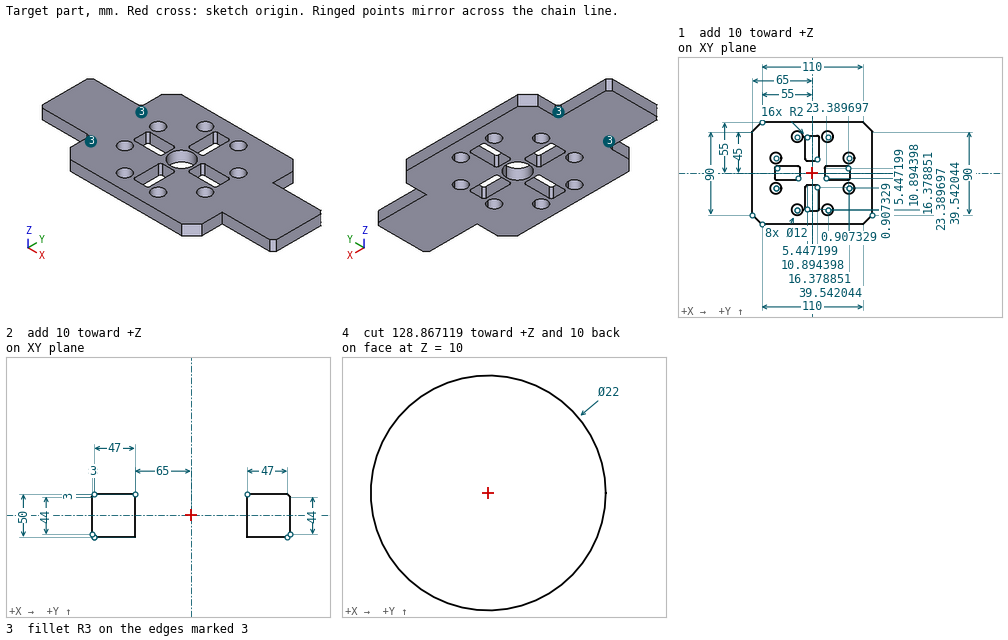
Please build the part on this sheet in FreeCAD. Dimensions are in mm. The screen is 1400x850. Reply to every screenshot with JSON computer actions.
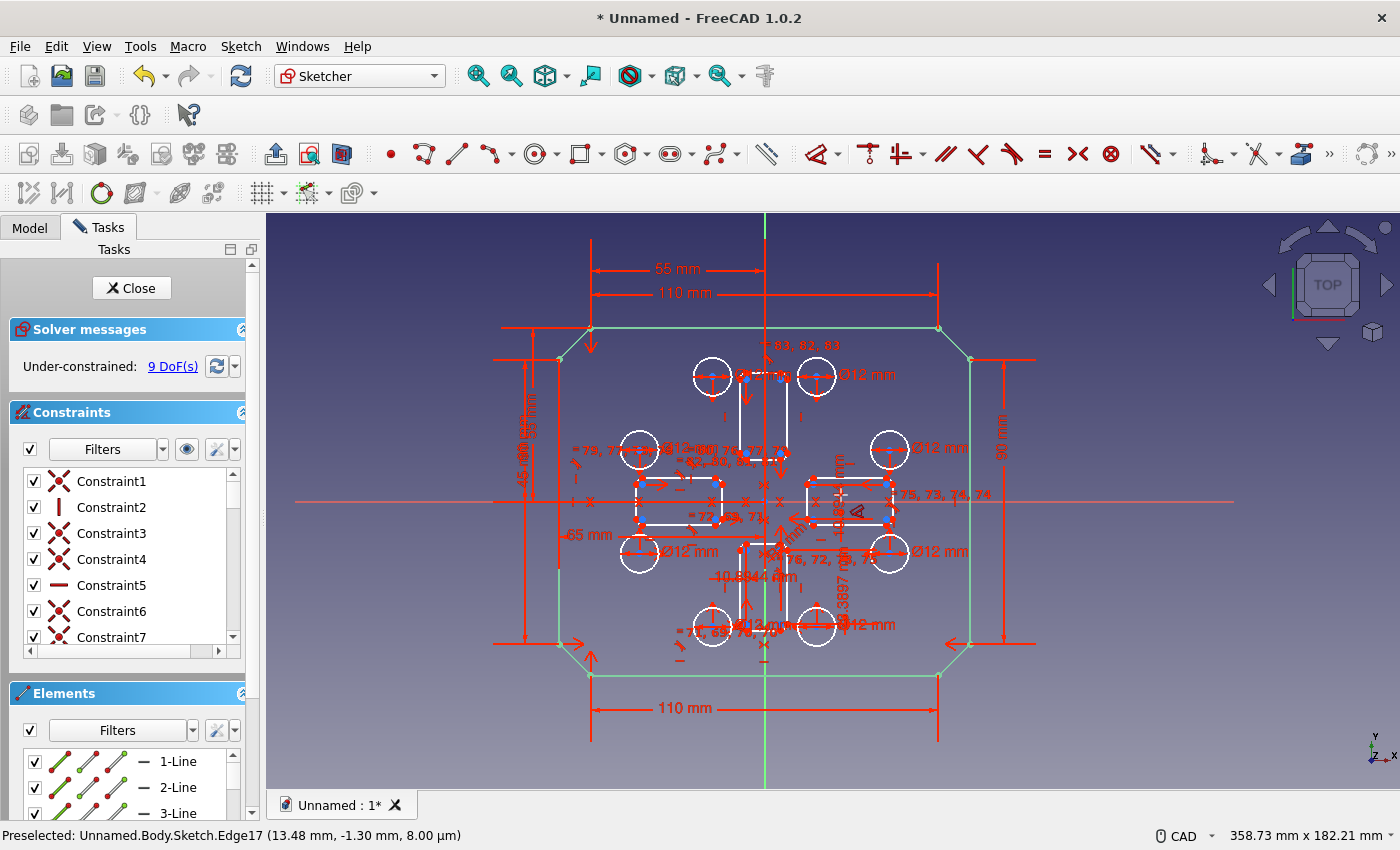
{"action": "left_click", "coordinate": [835, 478]}
{"action": "left_click", "coordinate": [850, 444]}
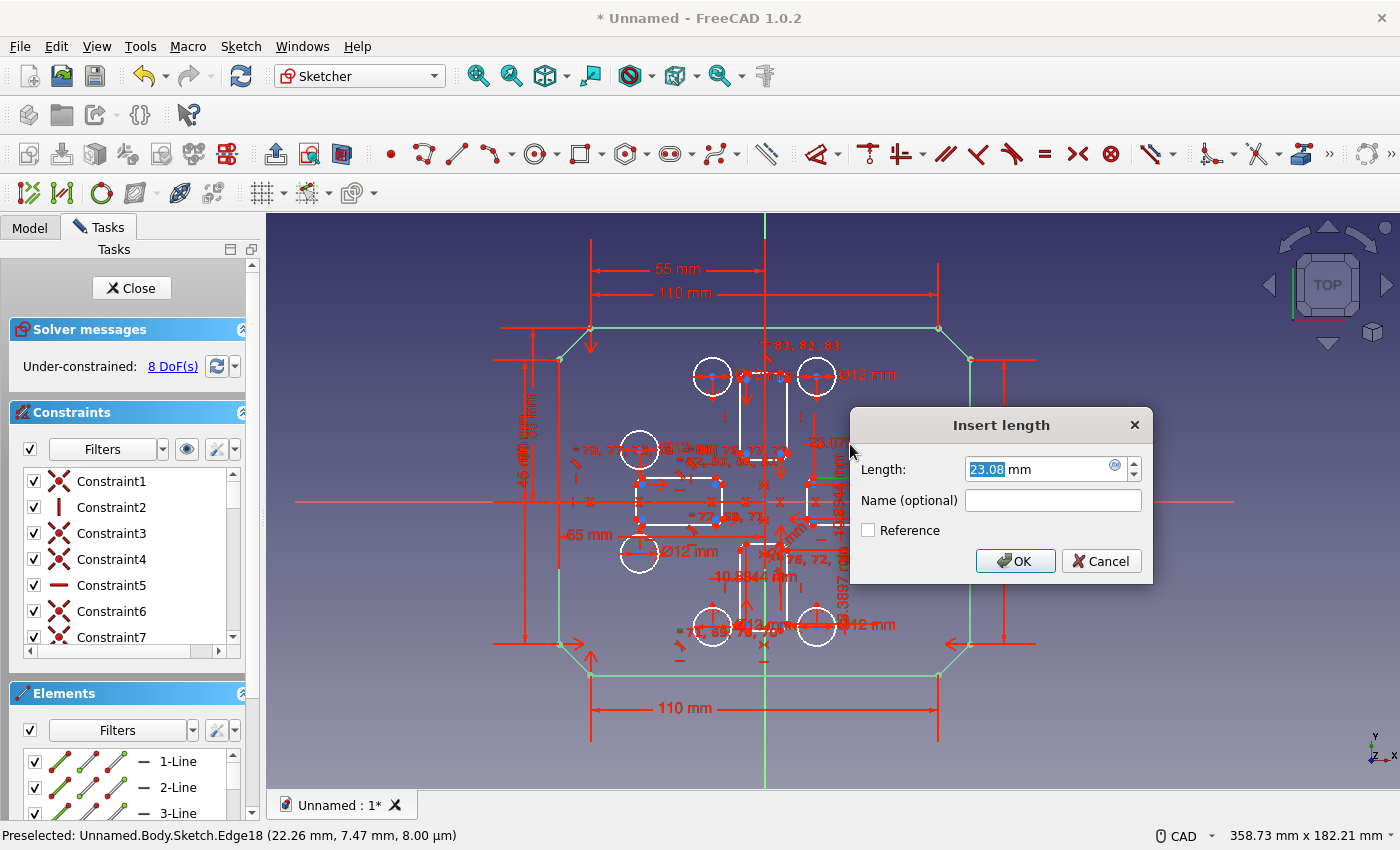
{"action": "type", "text": "23.389697"}
{"action": "key", "text": "Return"}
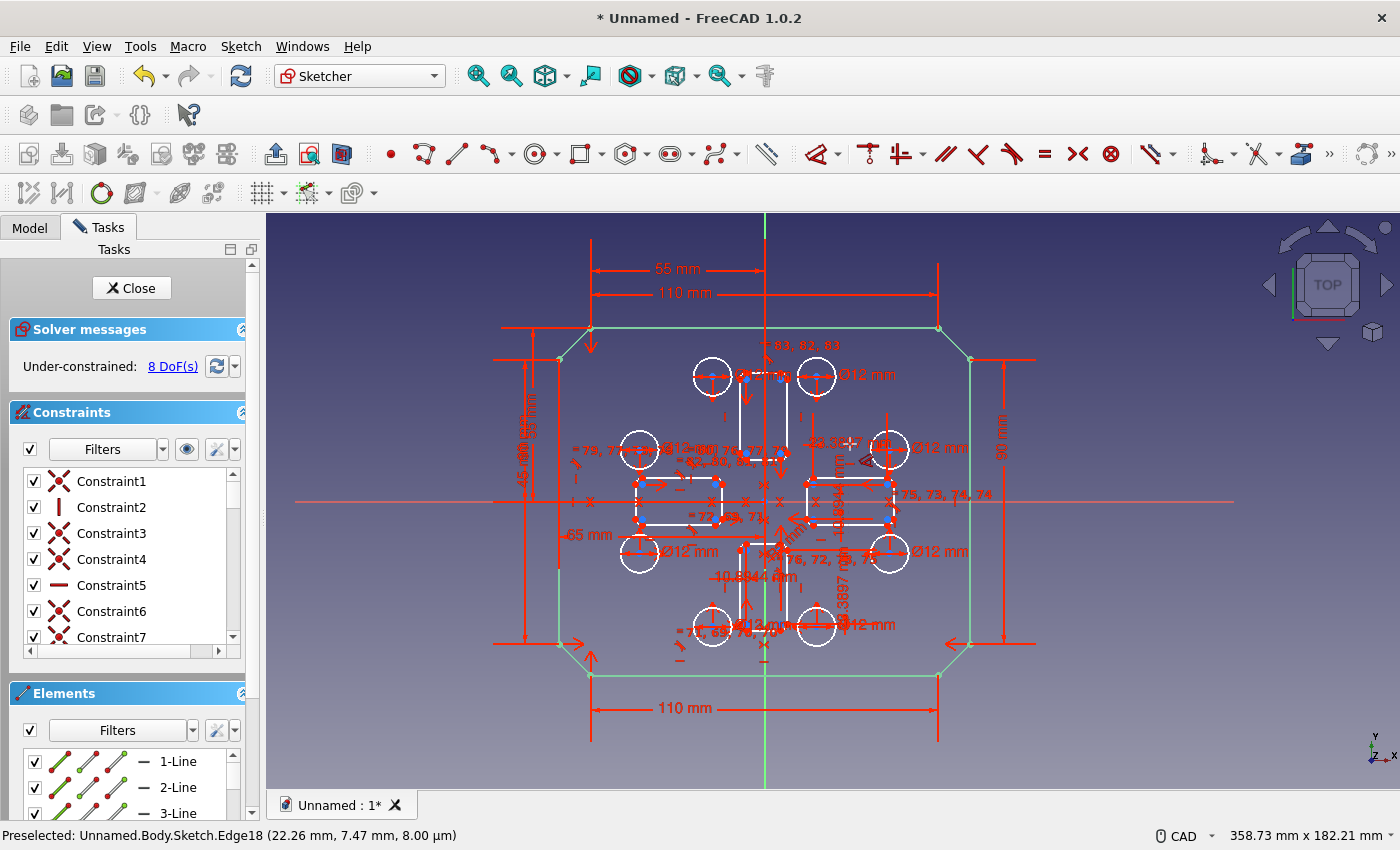
{"action": "scroll", "coordinate": [746, 544], "scroll_direction": "up", "scroll_amount": 5}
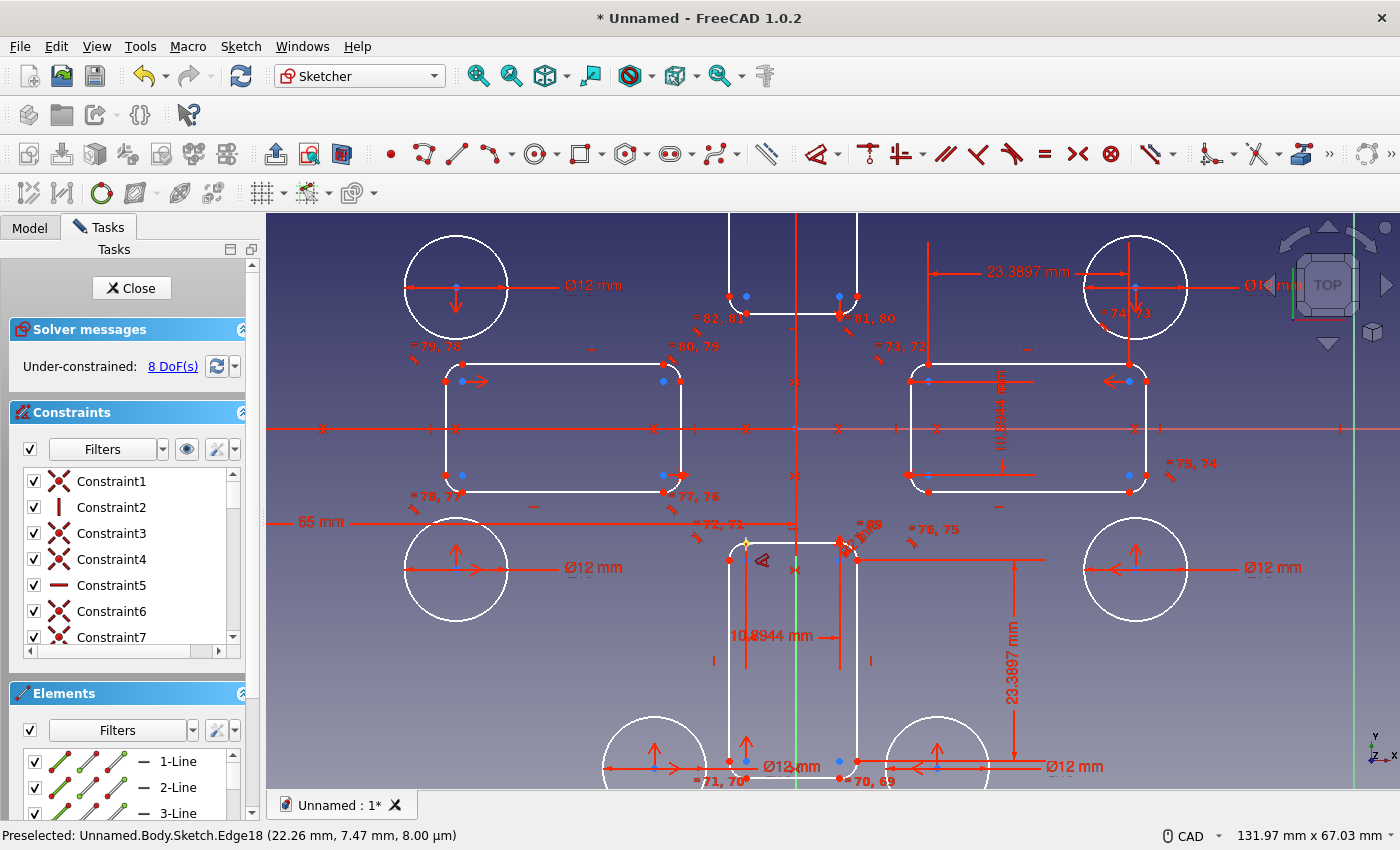
{"action": "left_click", "coordinate": [746, 543]}
{"action": "left_click", "coordinate": [771, 577]}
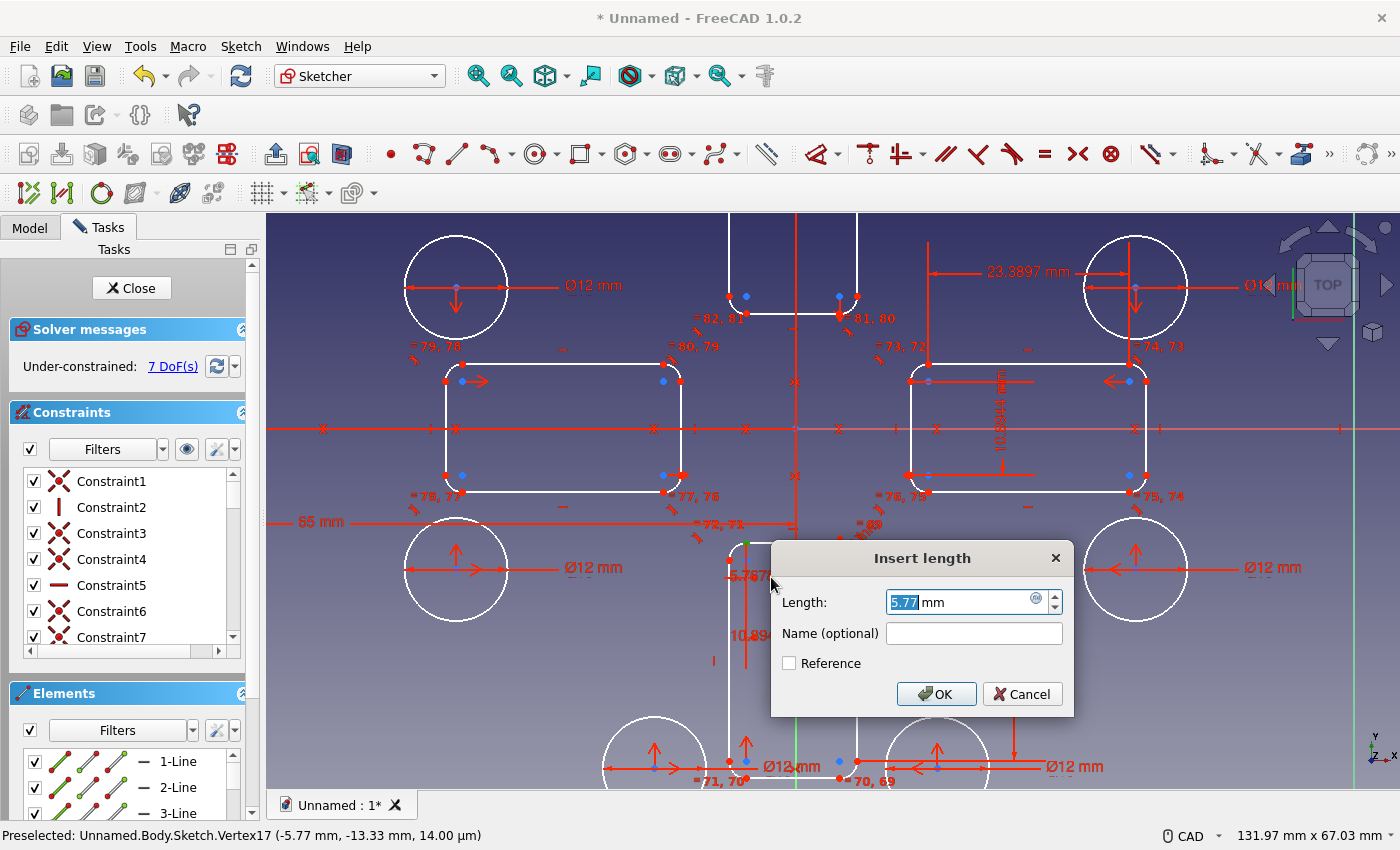
{"action": "type", "text": "5.447199"}
{"action": "key", "text": "Return"}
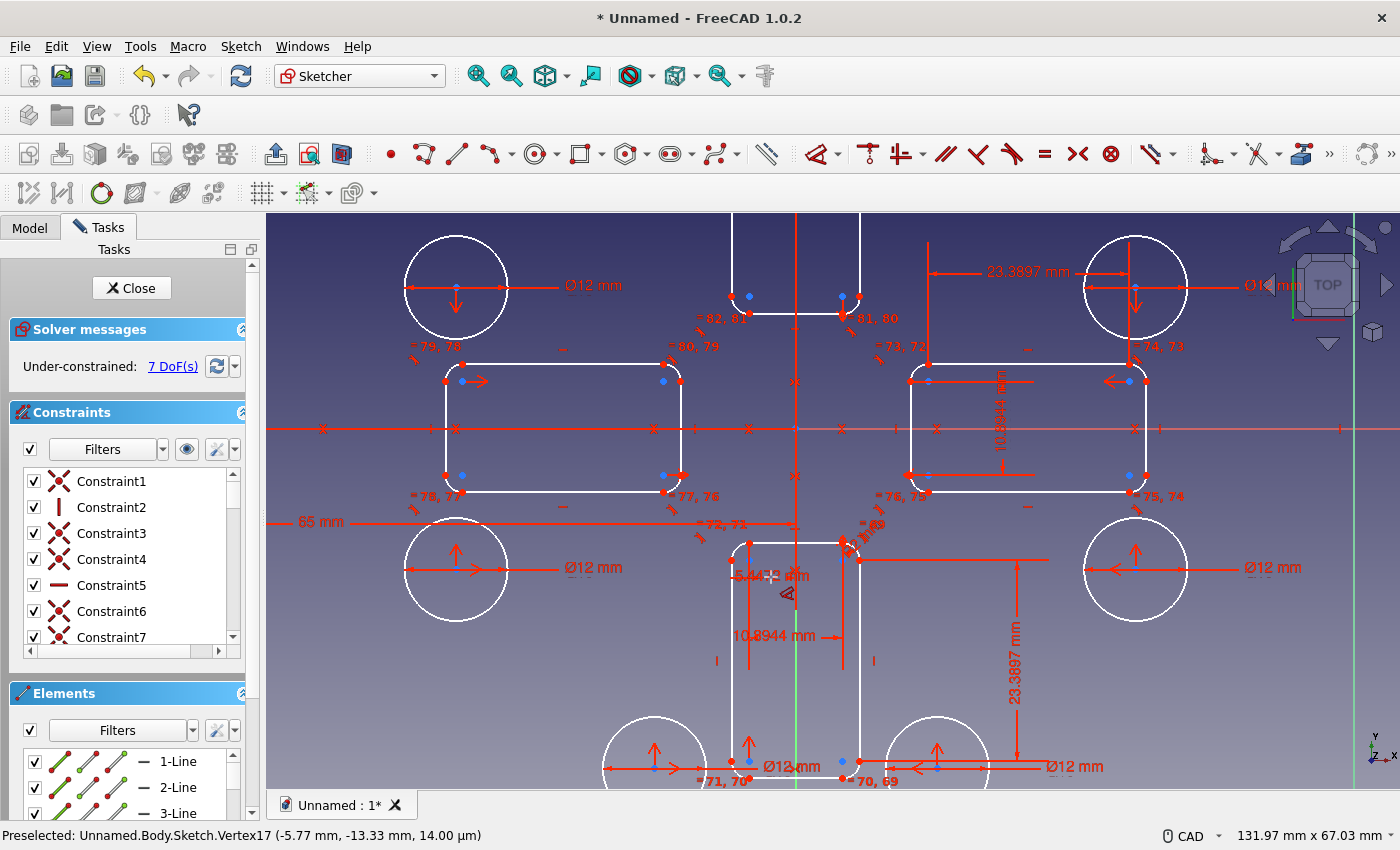
{"action": "left_click", "coordinate": [911, 475]}
{"action": "left_click", "coordinate": [945, 452]}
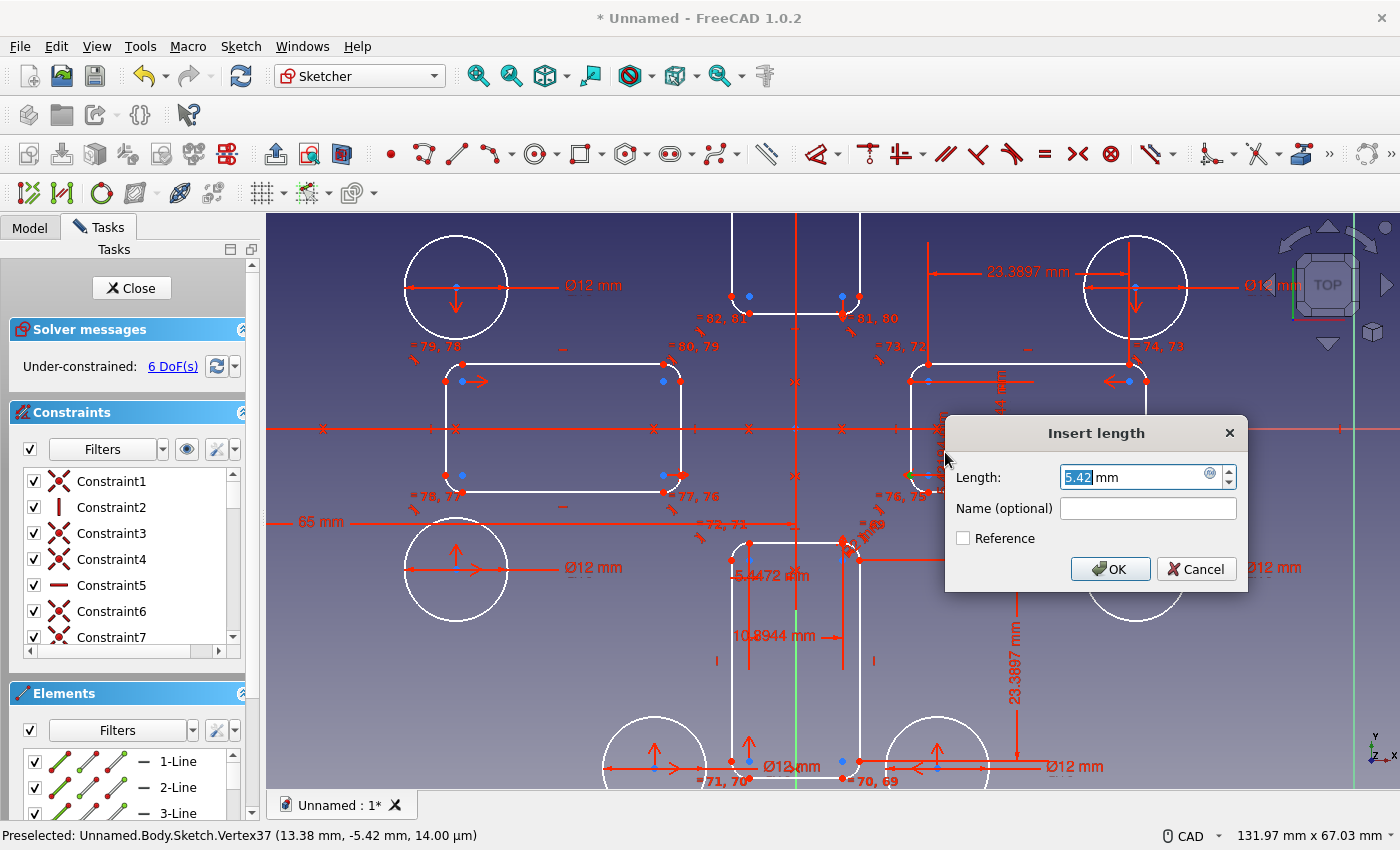
{"action": "type", "text": "5.447199"}
{"action": "key", "text": "Return"}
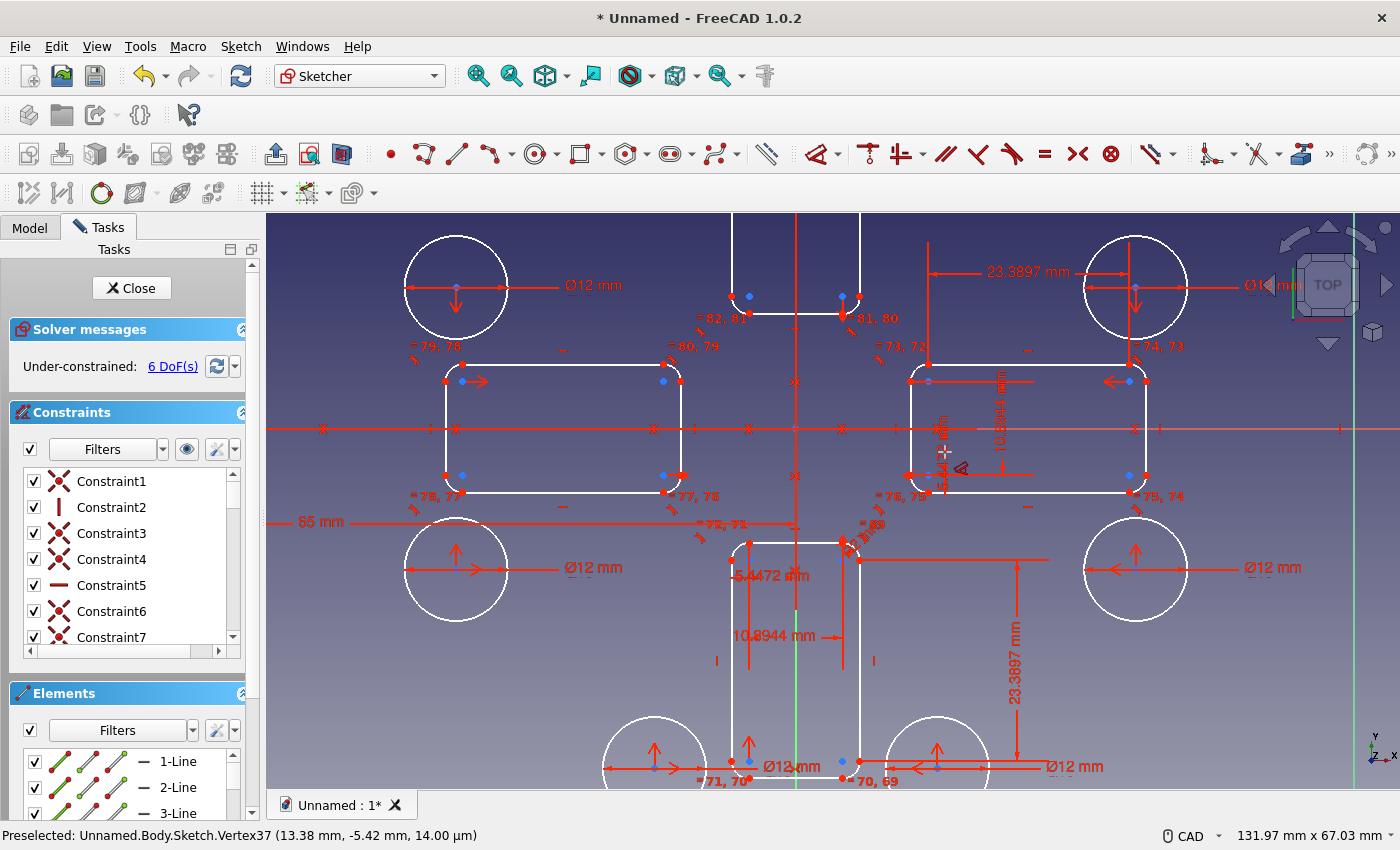
{"action": "scroll", "coordinate": [746, 543], "scroll_direction": "down", "scroll_amount": 5}